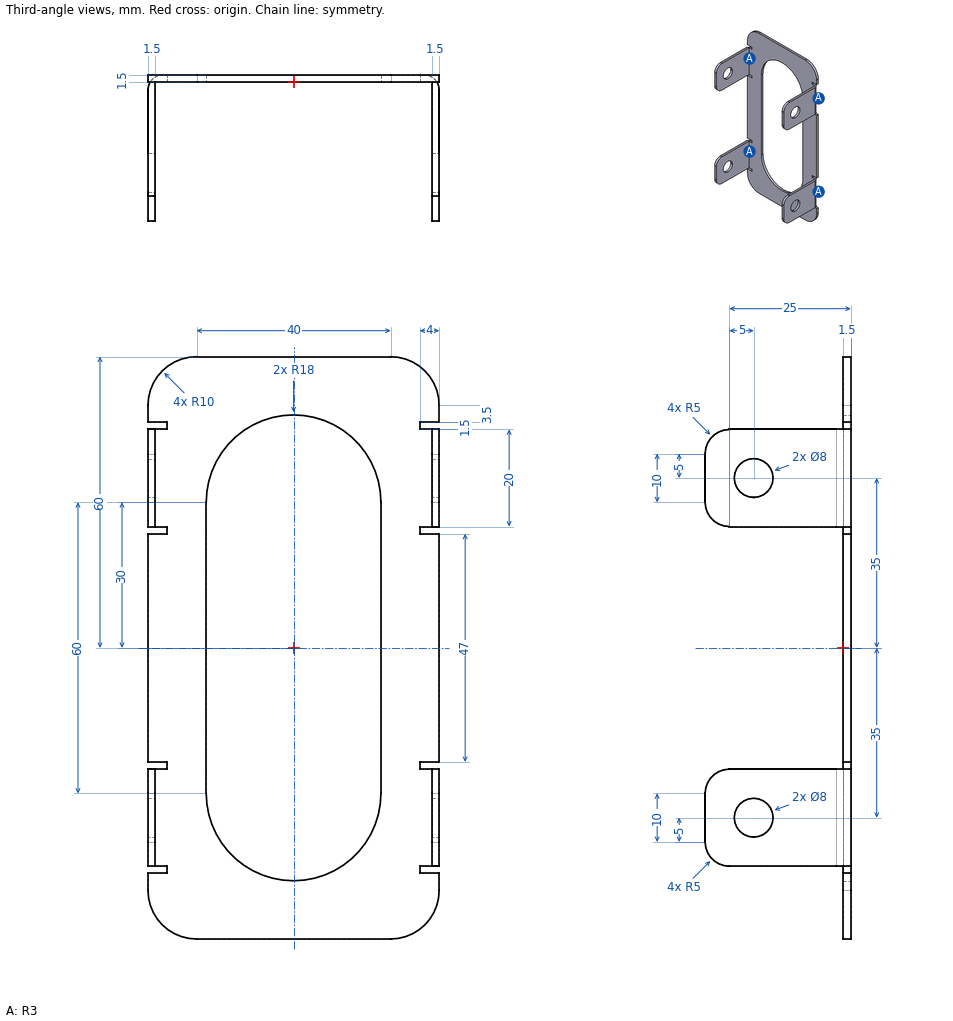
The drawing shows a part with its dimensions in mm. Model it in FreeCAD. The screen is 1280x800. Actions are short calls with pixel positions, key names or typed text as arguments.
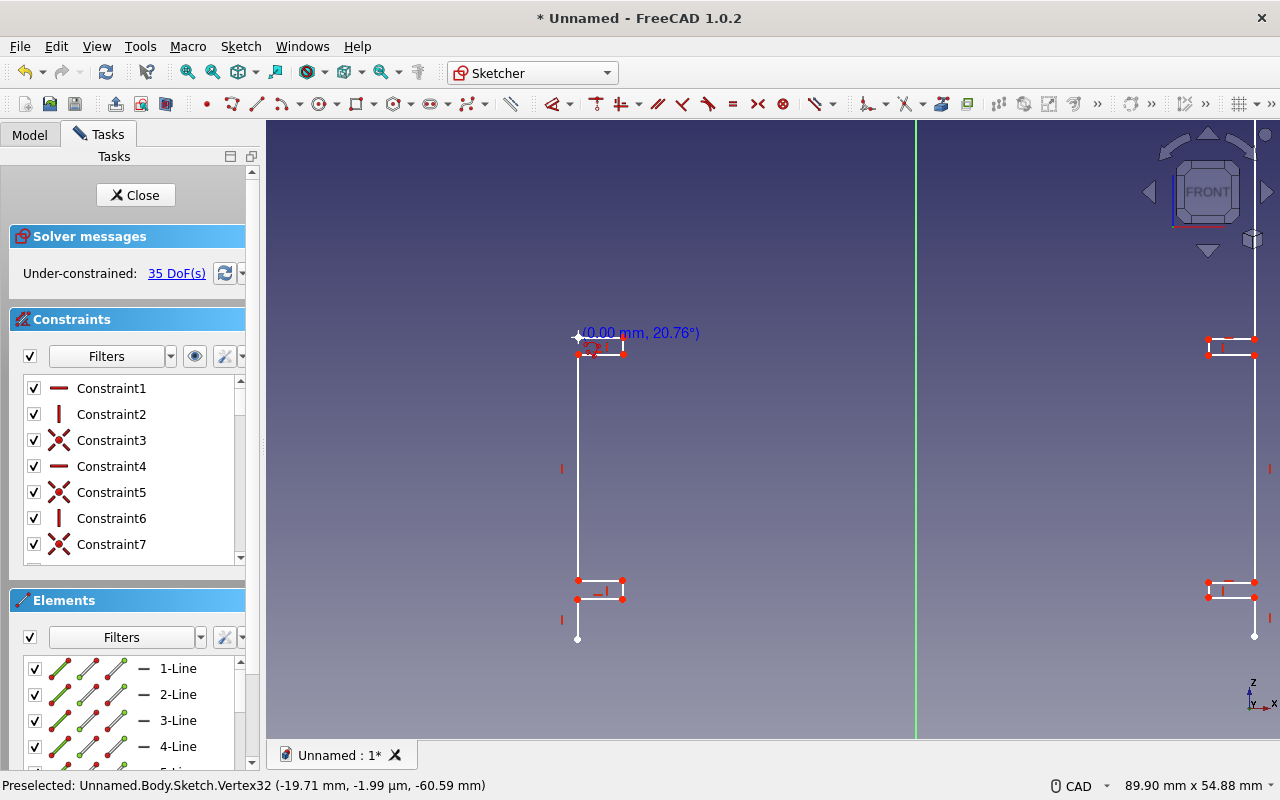
scroll(613, 584, down, 6)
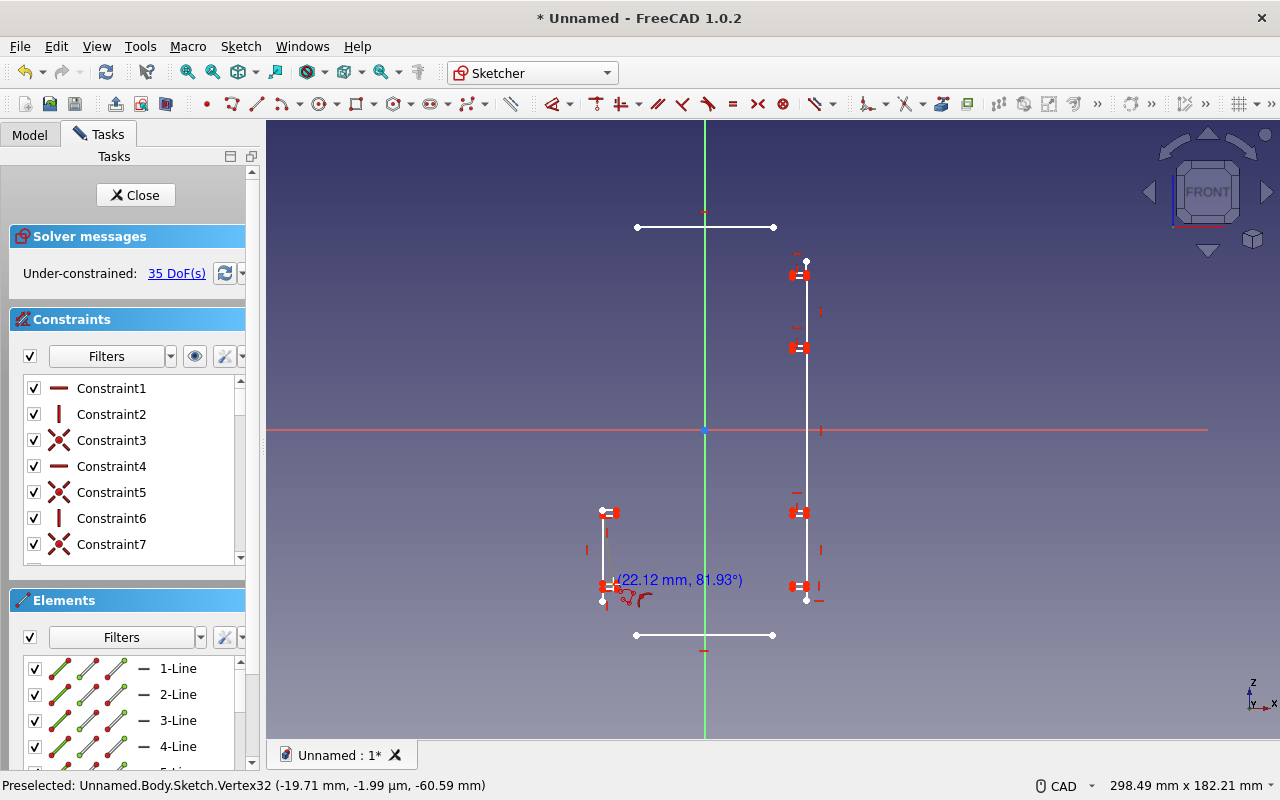
click(603, 350)
click(616, 350)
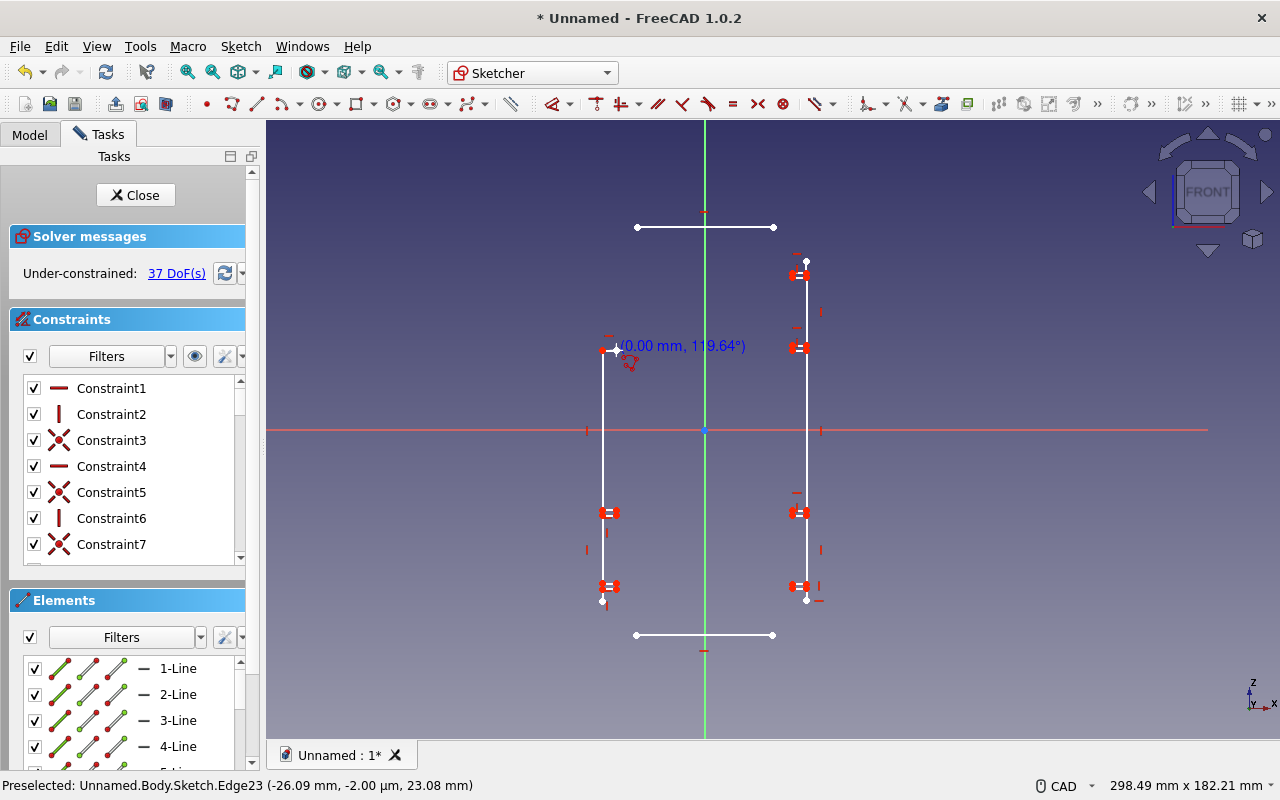
scroll(616, 345, up, 6)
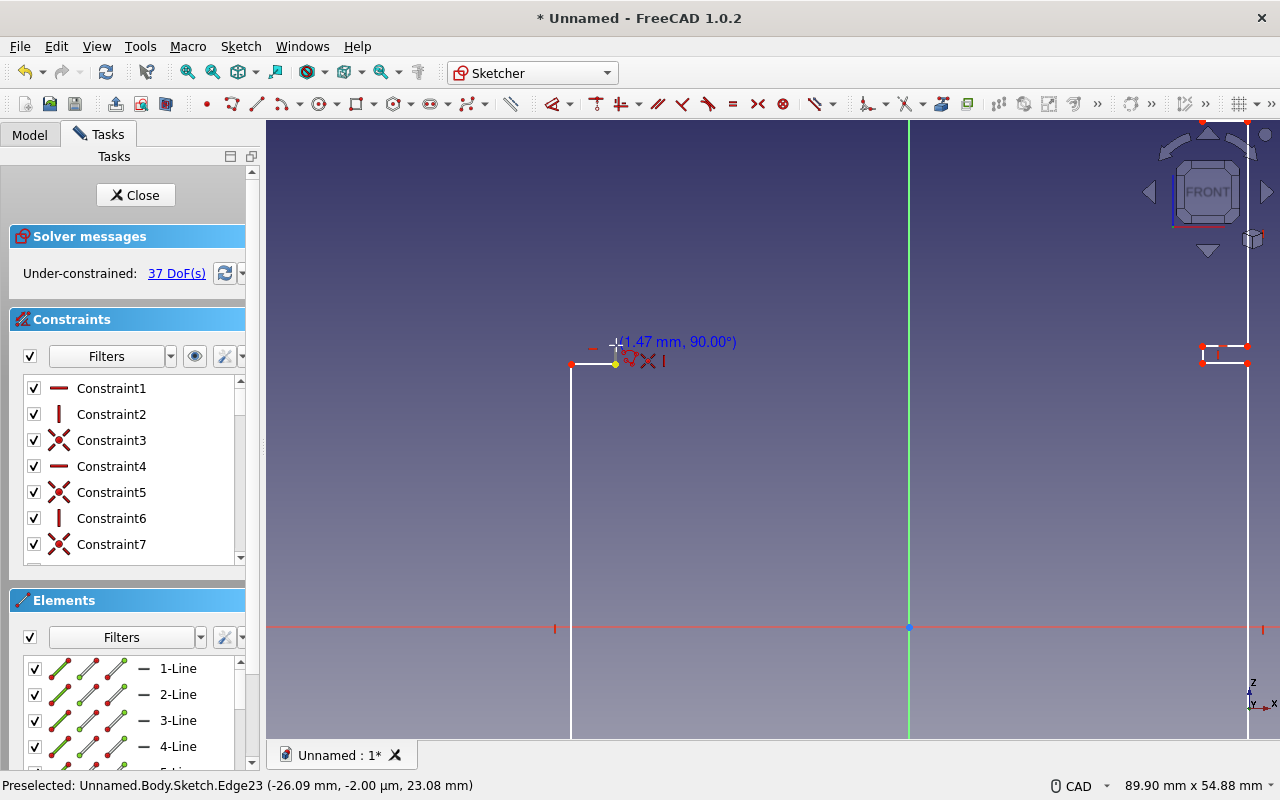
click(615, 345)
click(571, 345)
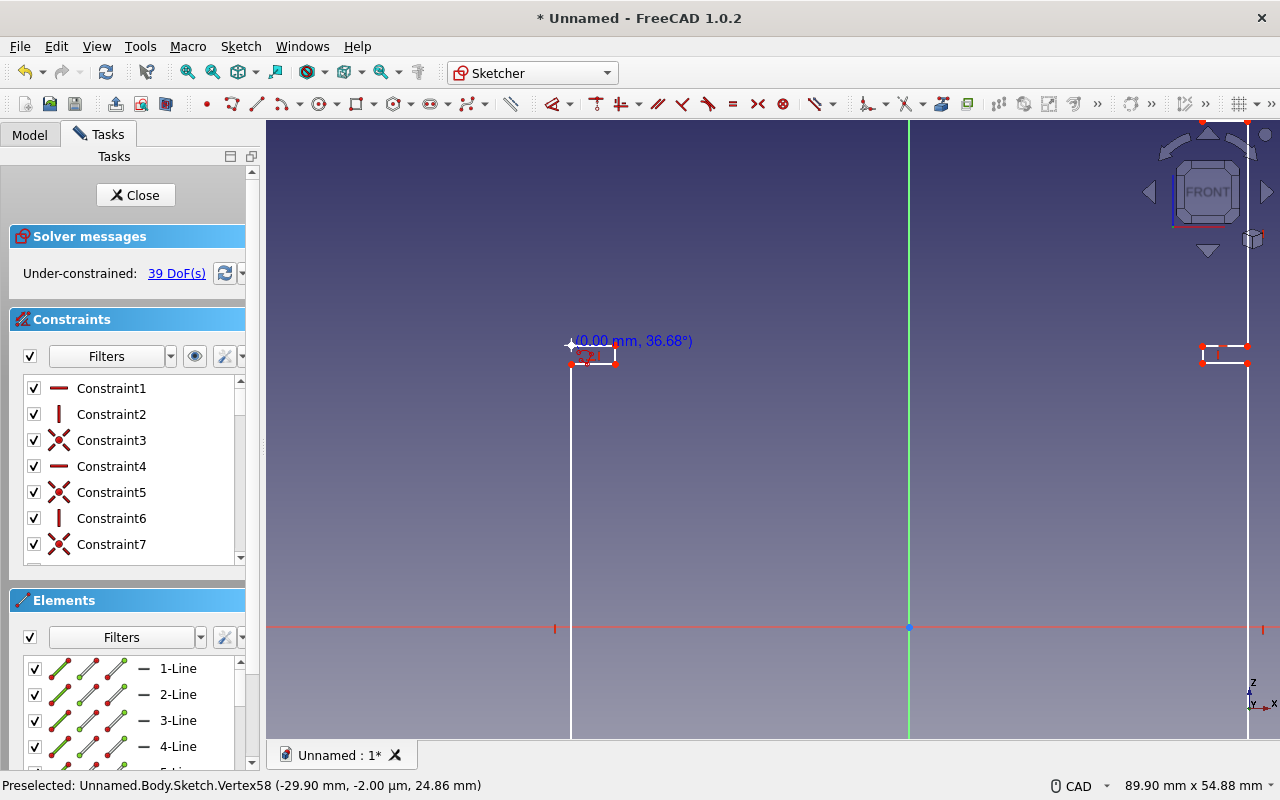
scroll(616, 344, down, 6)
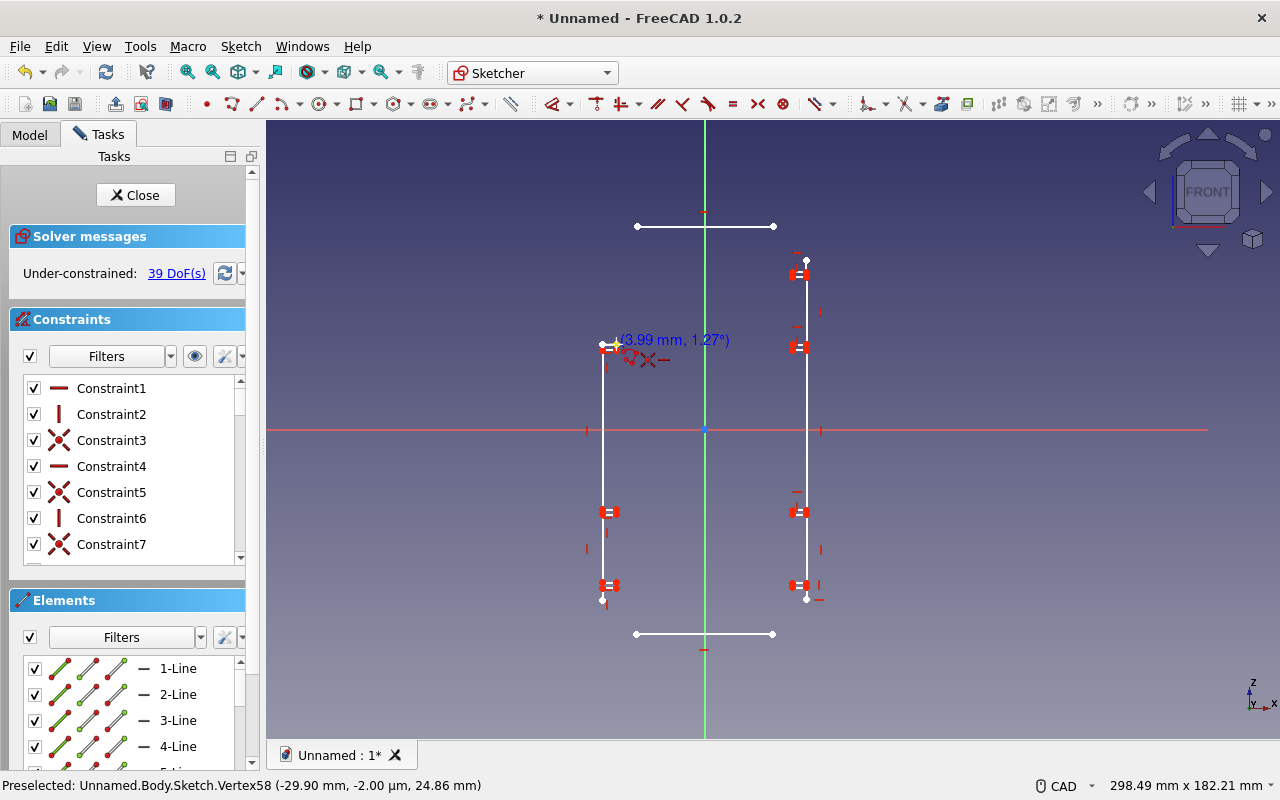
click(603, 277)
click(616, 277)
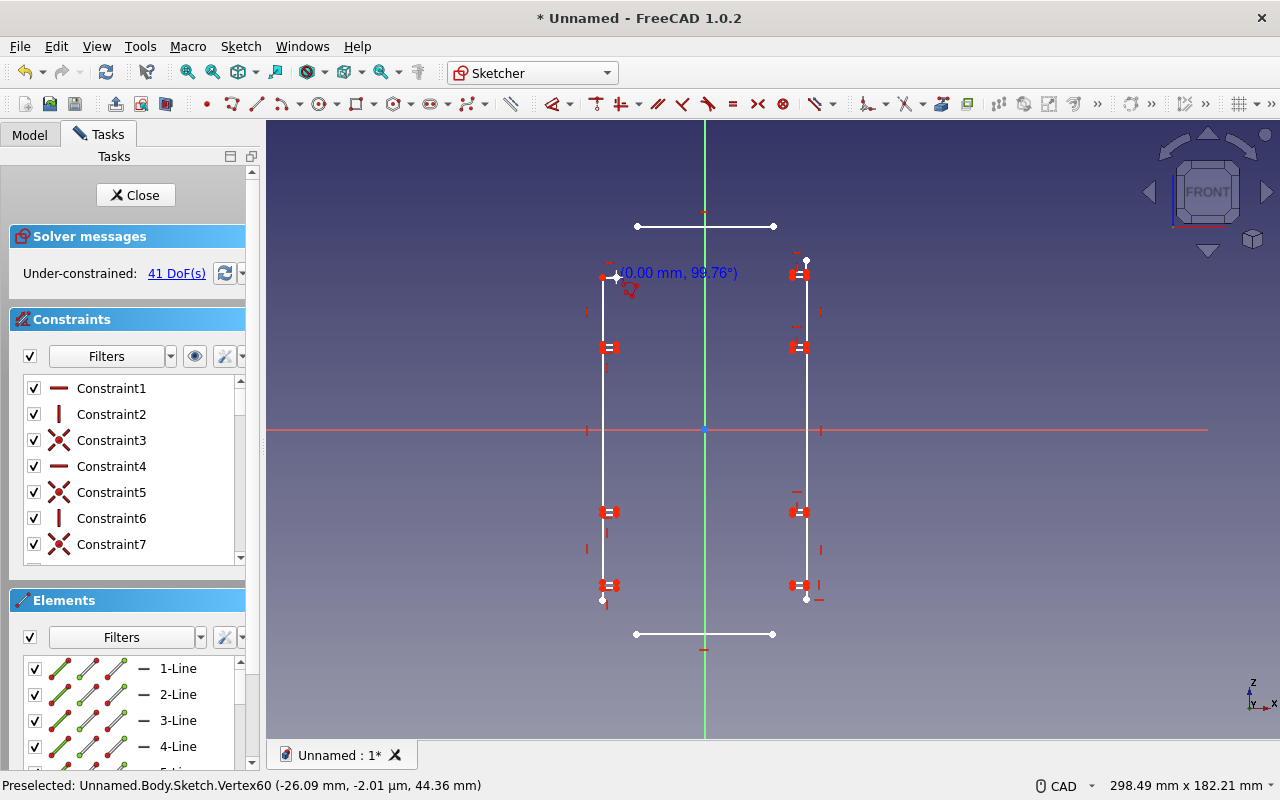
scroll(616, 272, up, 6)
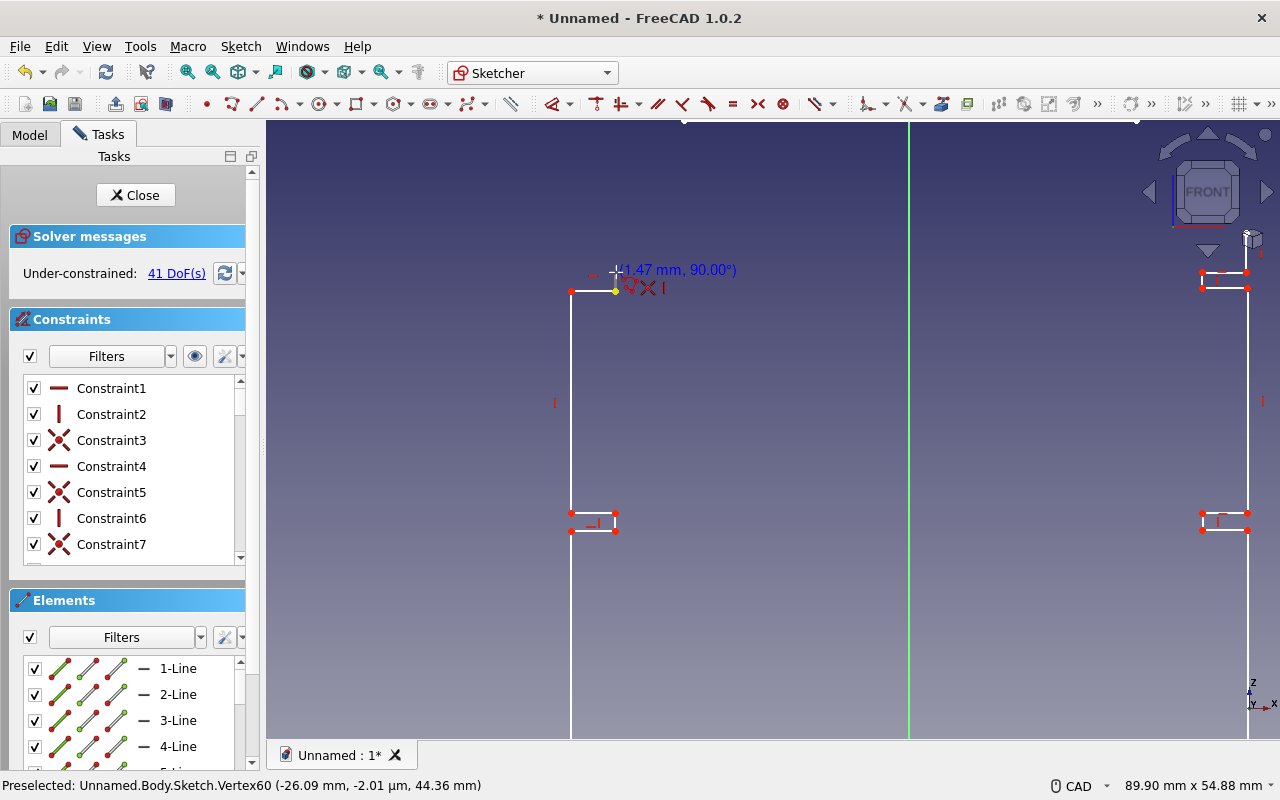
click(615, 270)
click(571, 270)
click(571, 231)
right_click(571, 231)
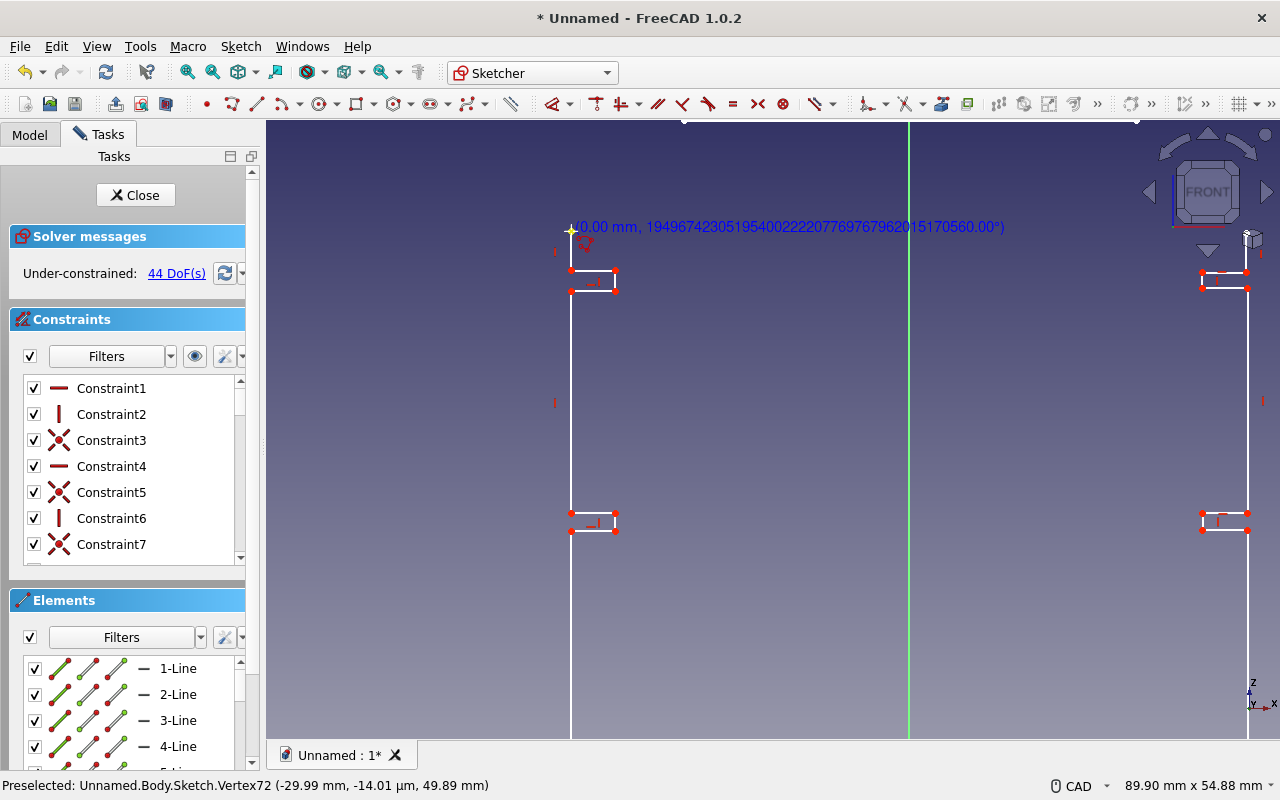
click(300, 104)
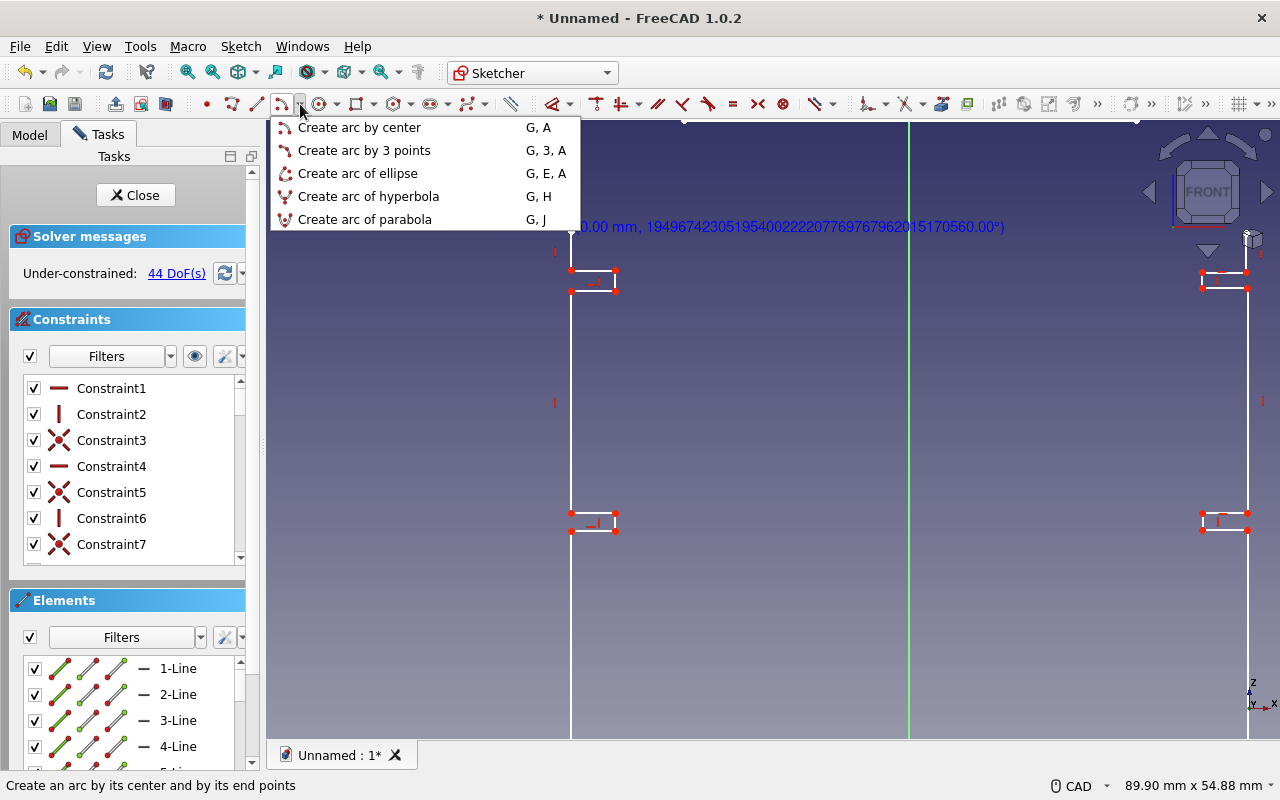
click(426, 150)